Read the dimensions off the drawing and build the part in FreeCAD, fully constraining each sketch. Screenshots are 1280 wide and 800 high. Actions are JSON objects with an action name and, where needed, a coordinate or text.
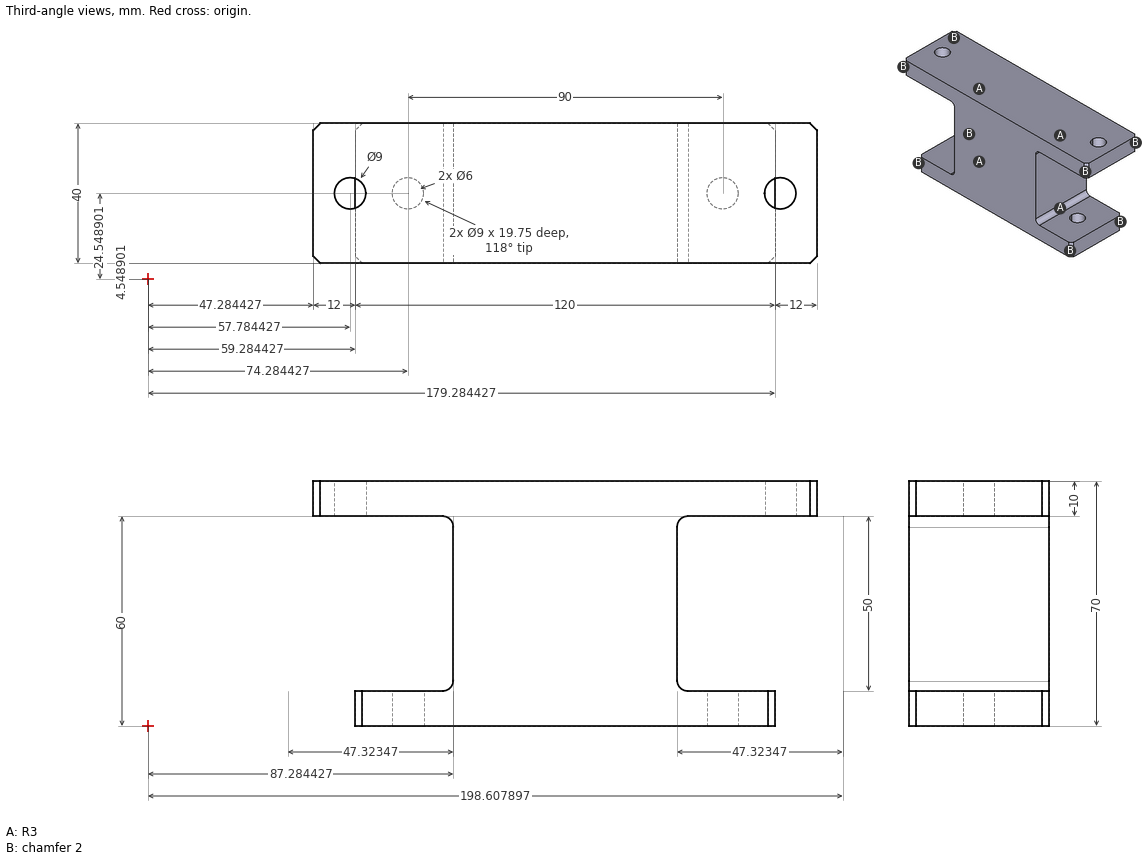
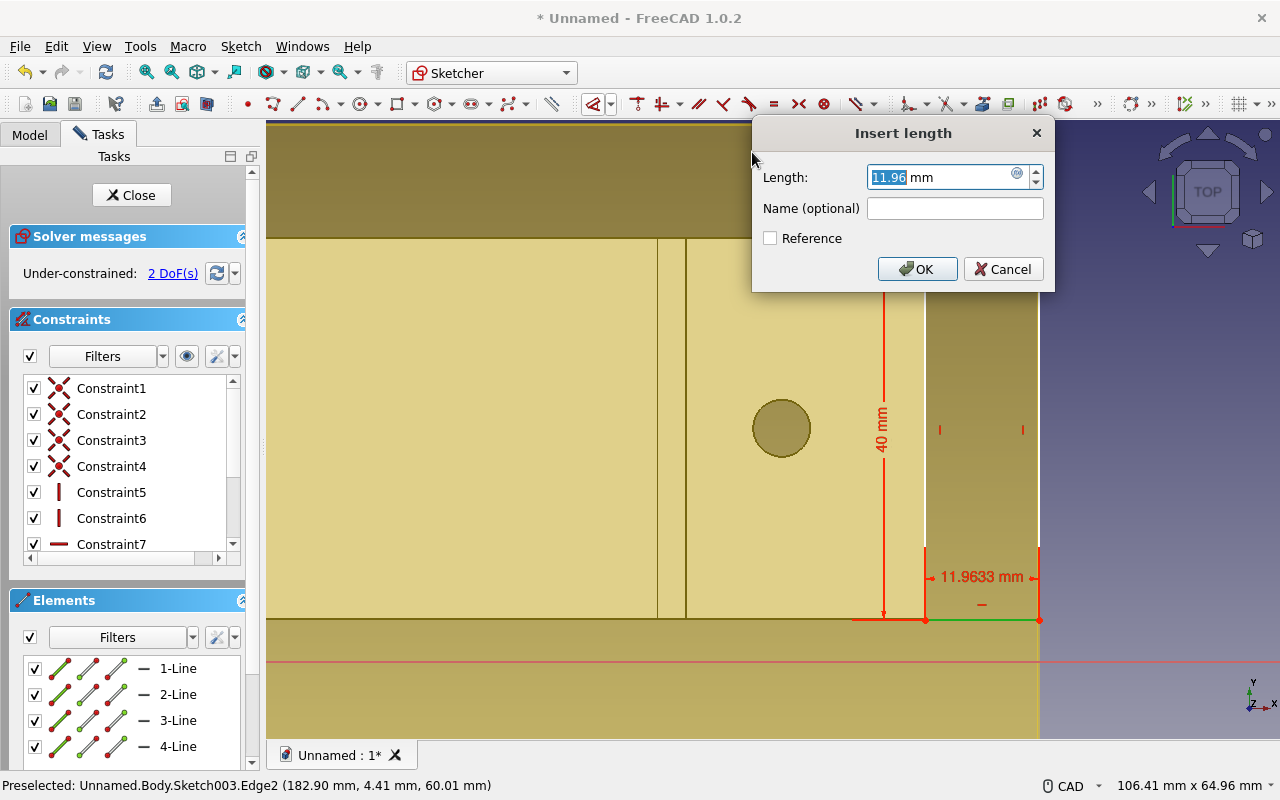
{"action": "type", "text": "12"}
{"action": "key", "text": "Return"}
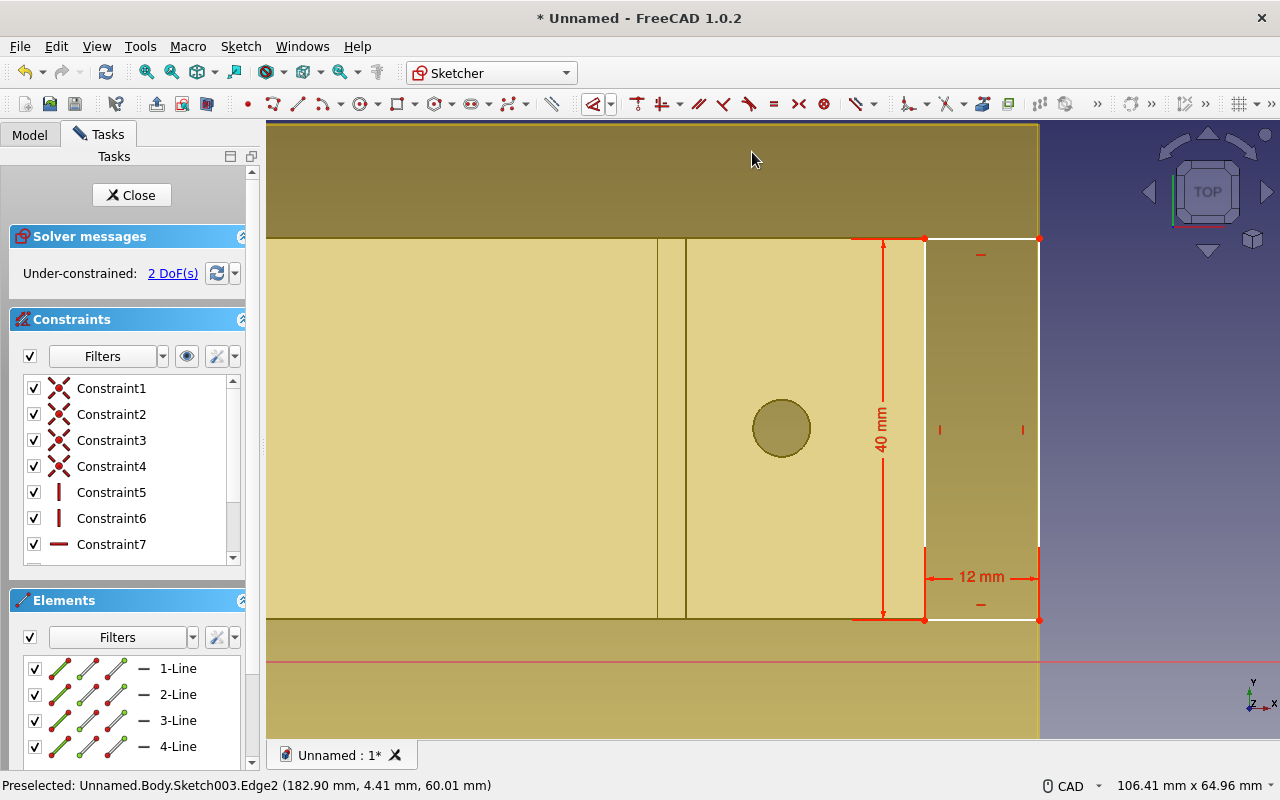
{"action": "left_click", "coordinate": [925, 620]}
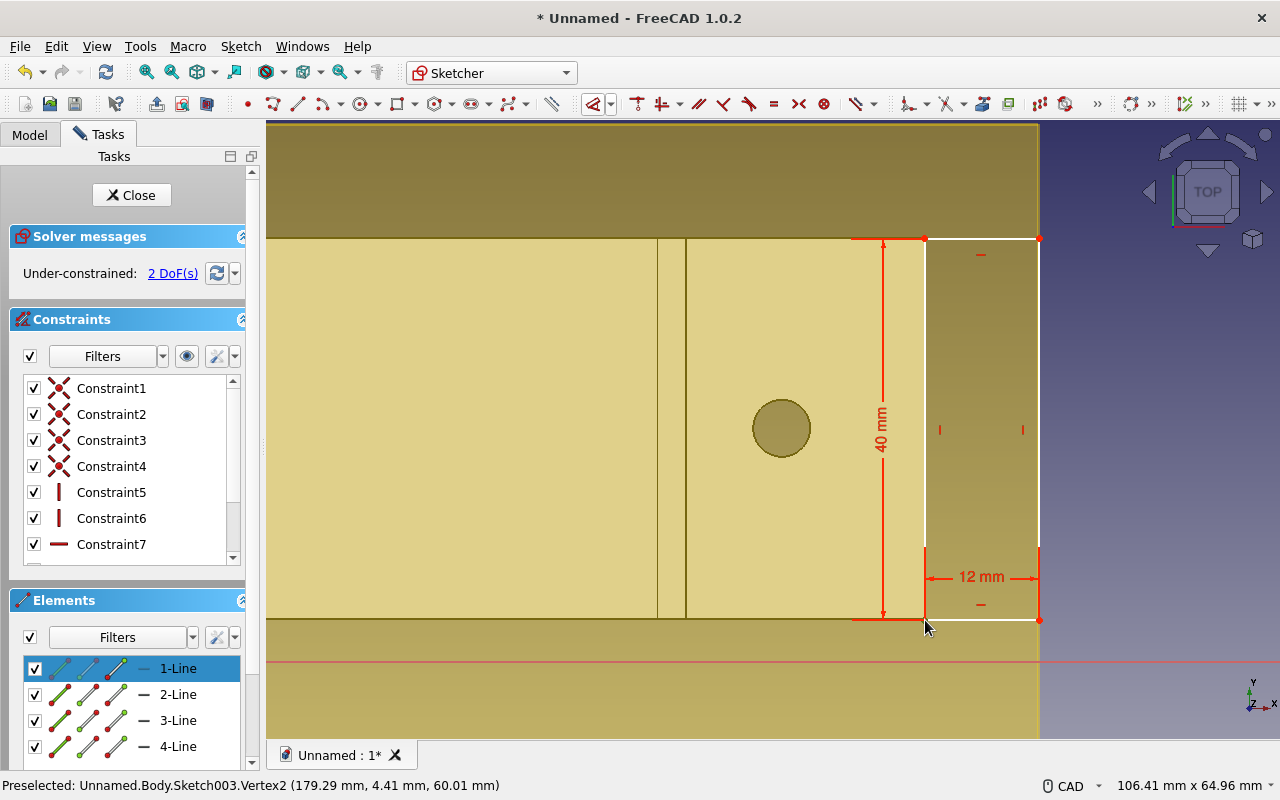
{"action": "key", "text": "i"}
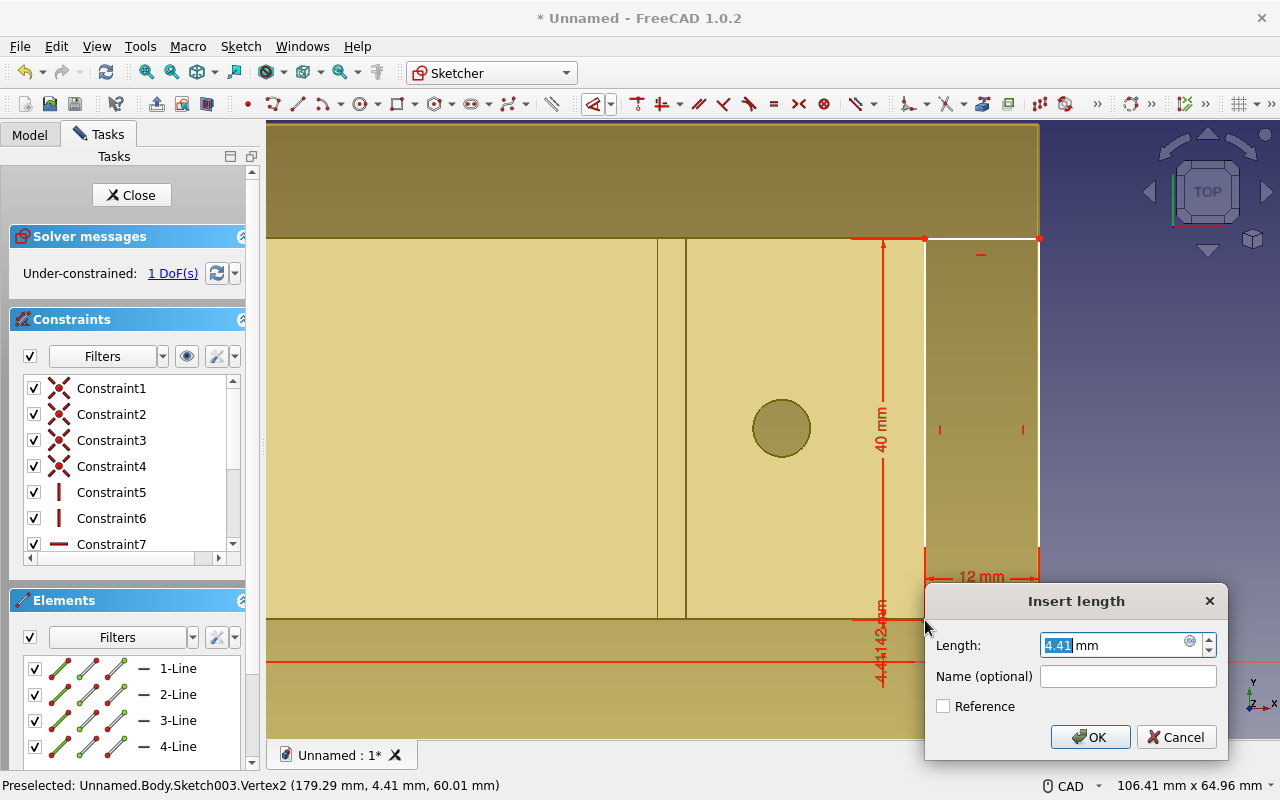
{"action": "type", "text": "4.548901"}
{"action": "key", "text": "Return"}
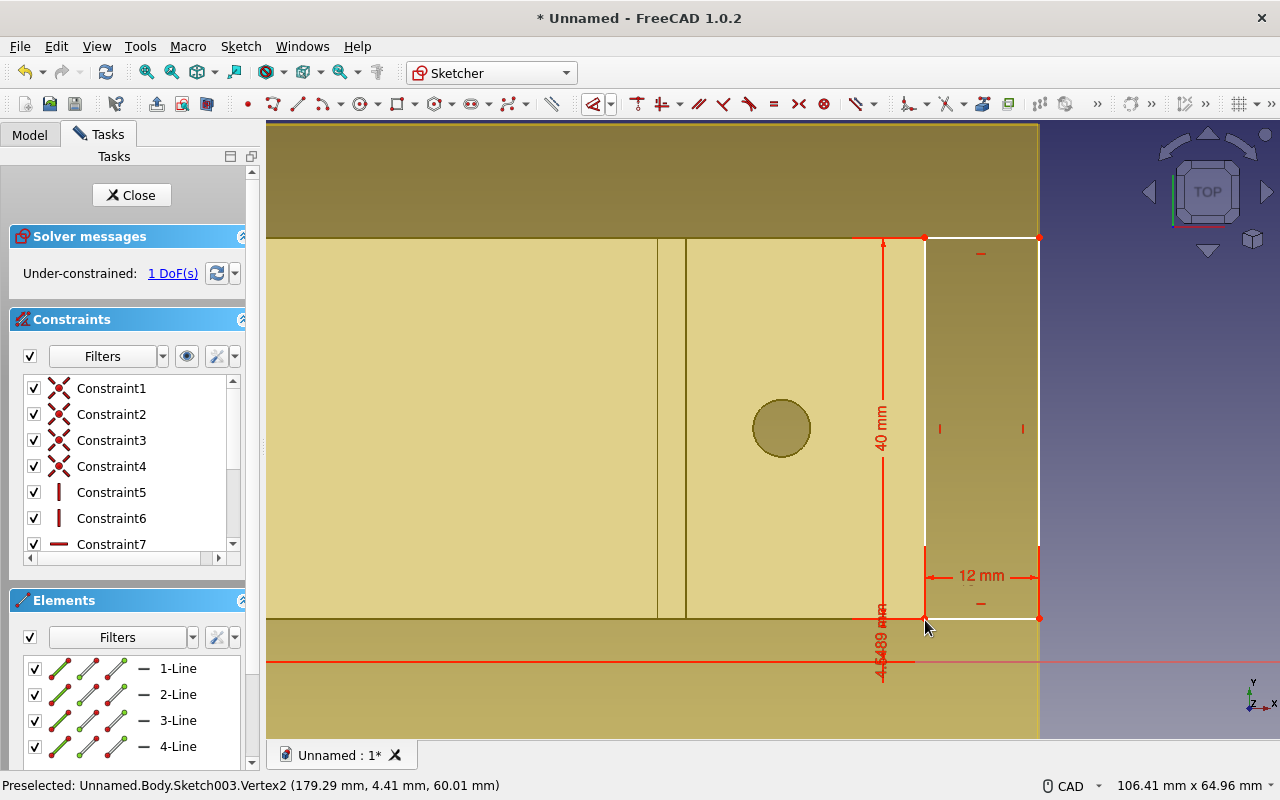
{"action": "left_click", "coordinate": [925, 238]}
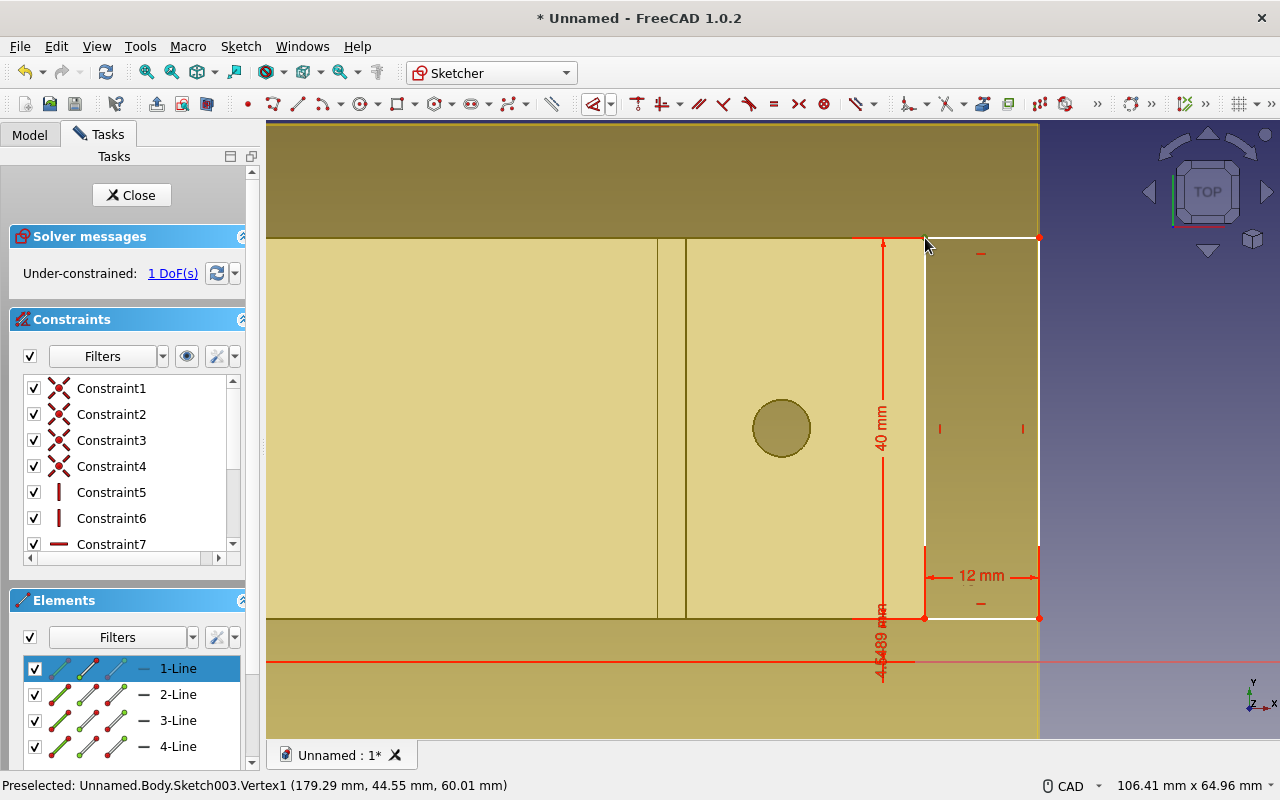
{"action": "key", "text": "l"}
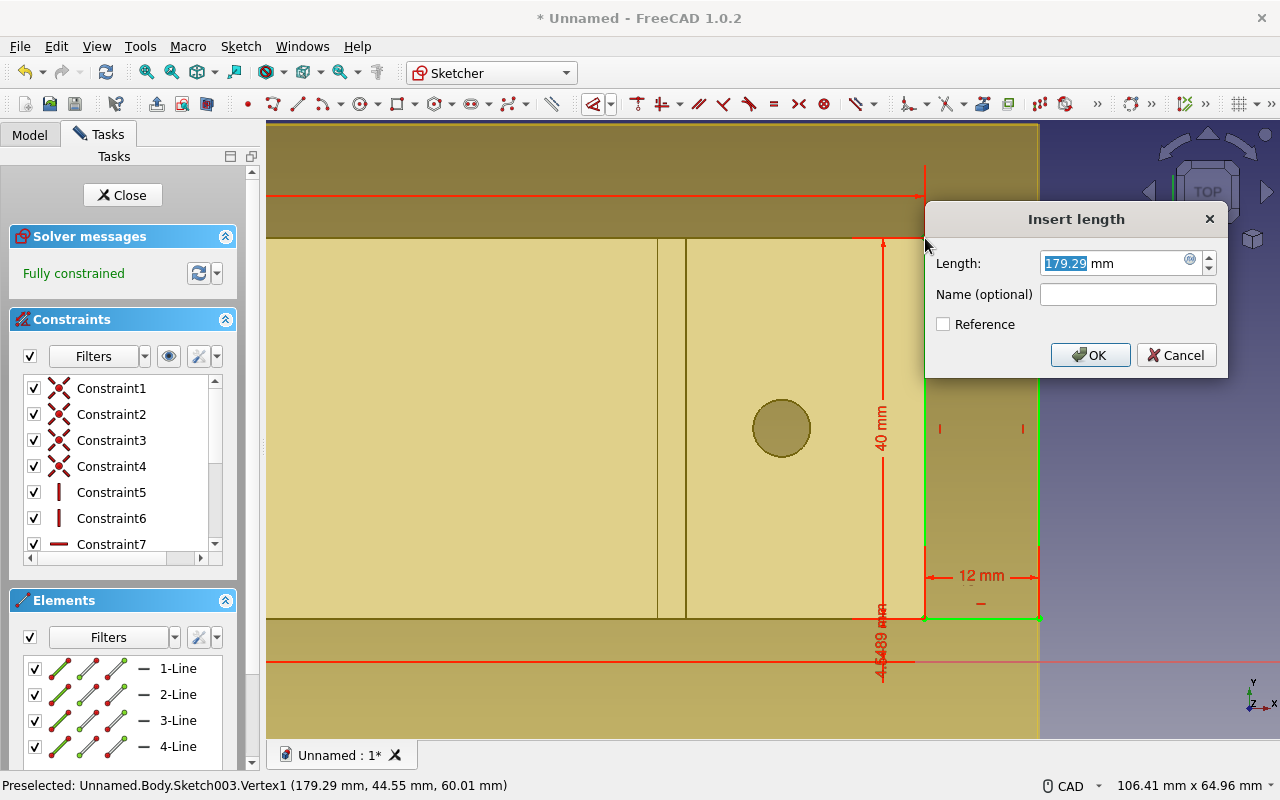
{"action": "type", "text": "179.284427"}
{"action": "key", "text": "Return"}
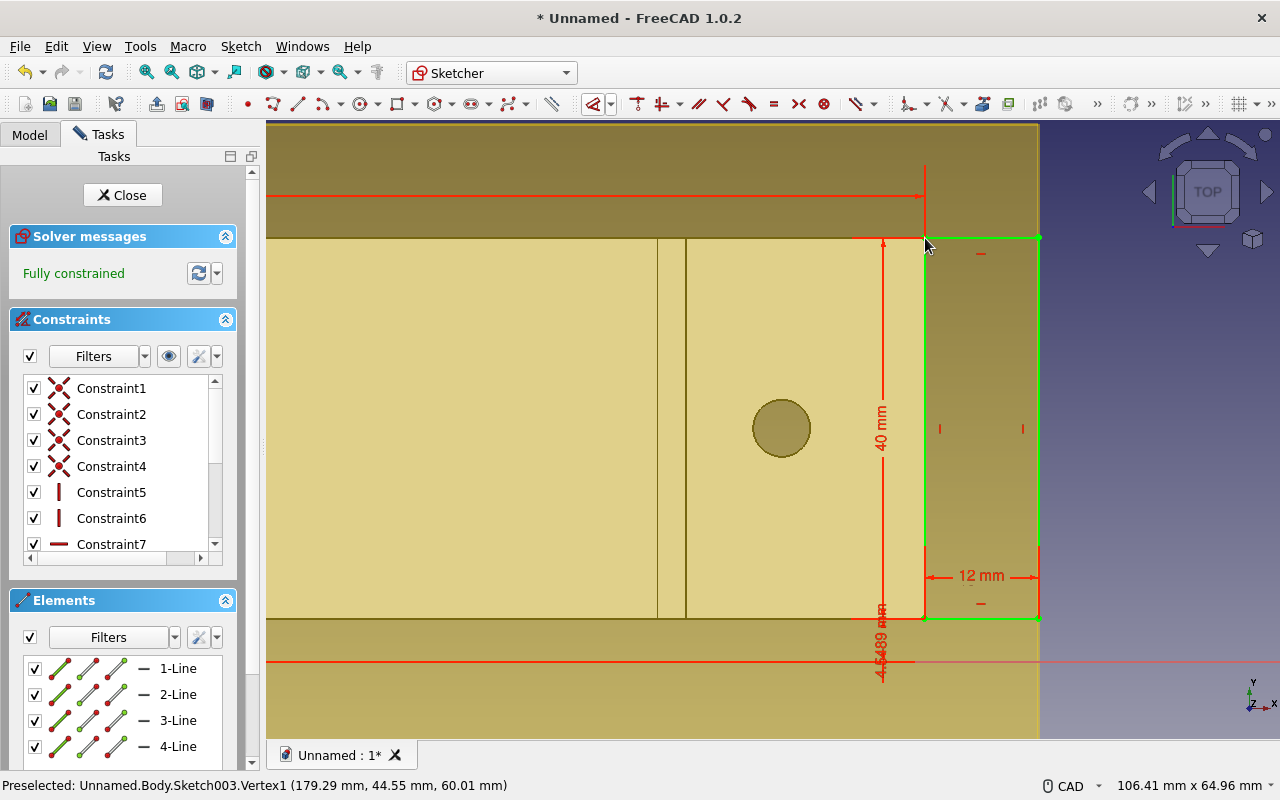
{"action": "left_click", "coordinate": [123, 195]}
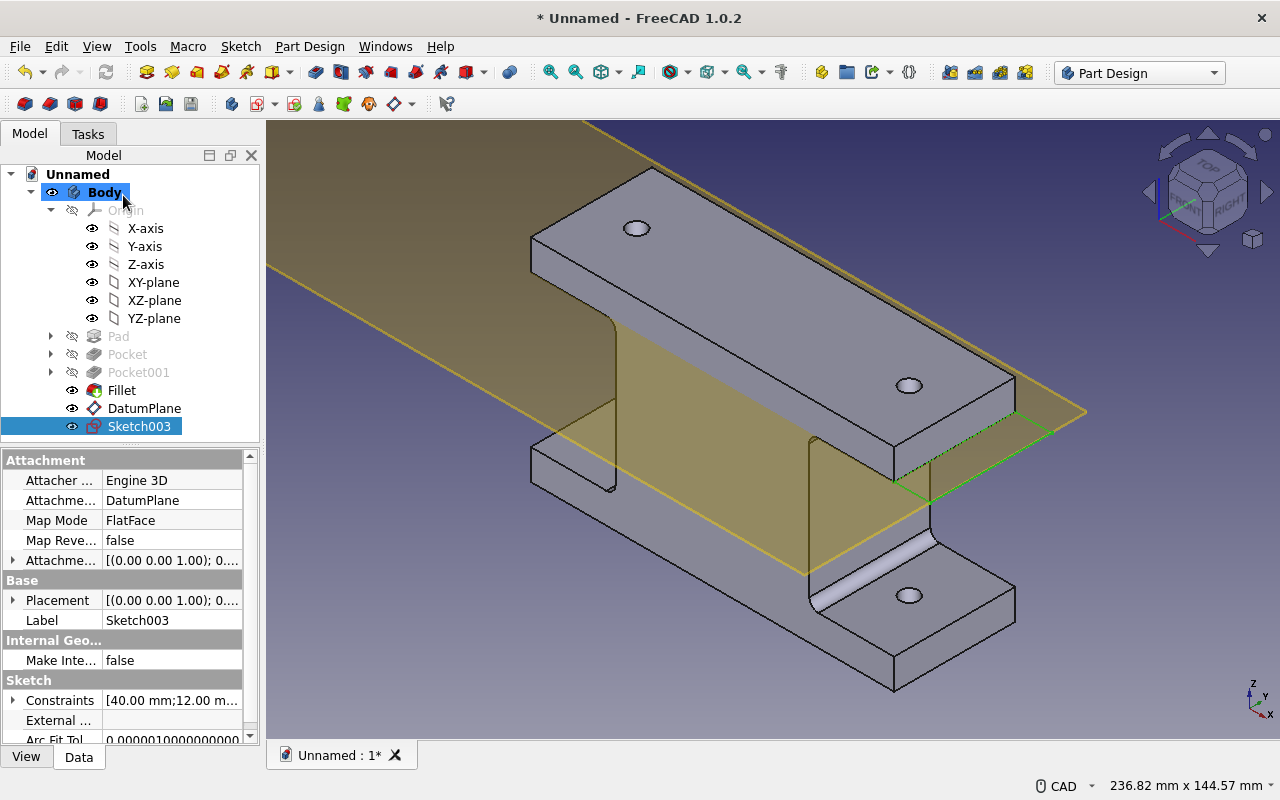
{"action": "left_click", "coordinate": [147, 72]}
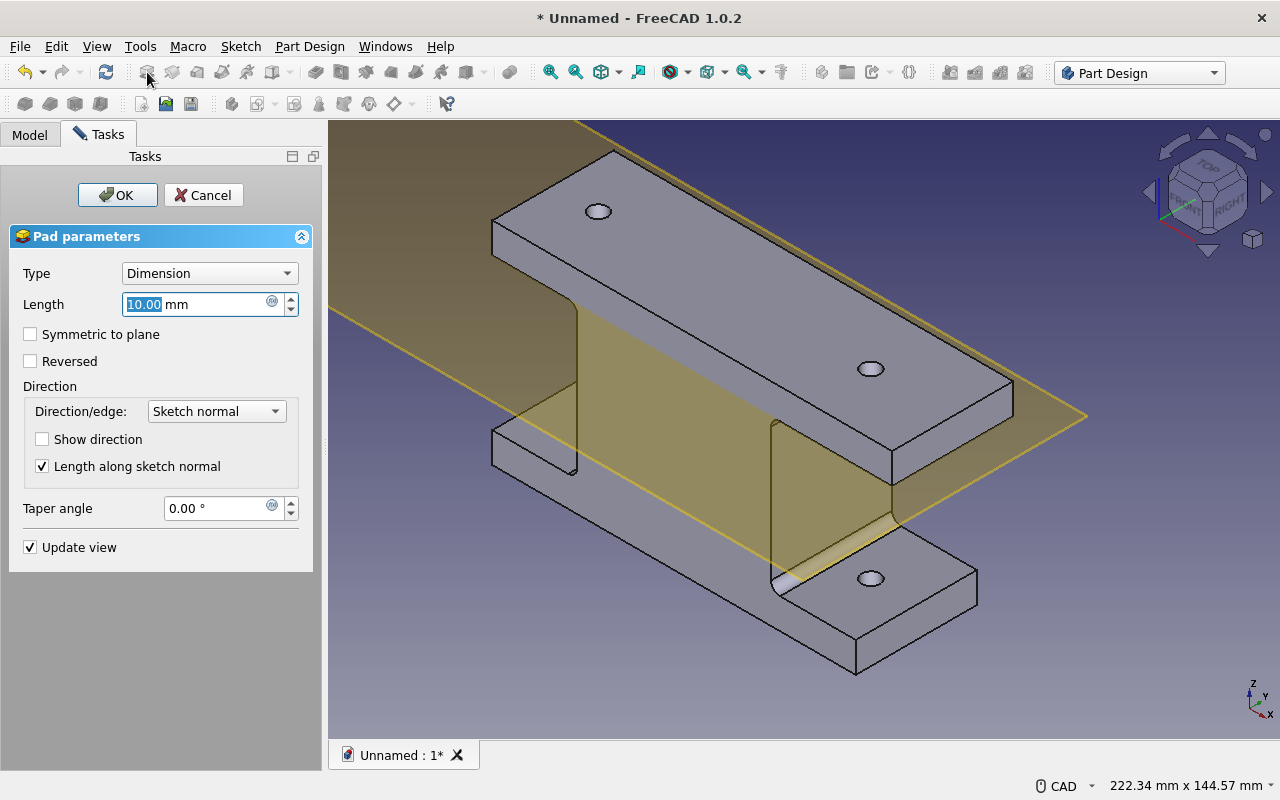
{"action": "type", "text": "10"}
{"action": "key", "text": "Tab"}